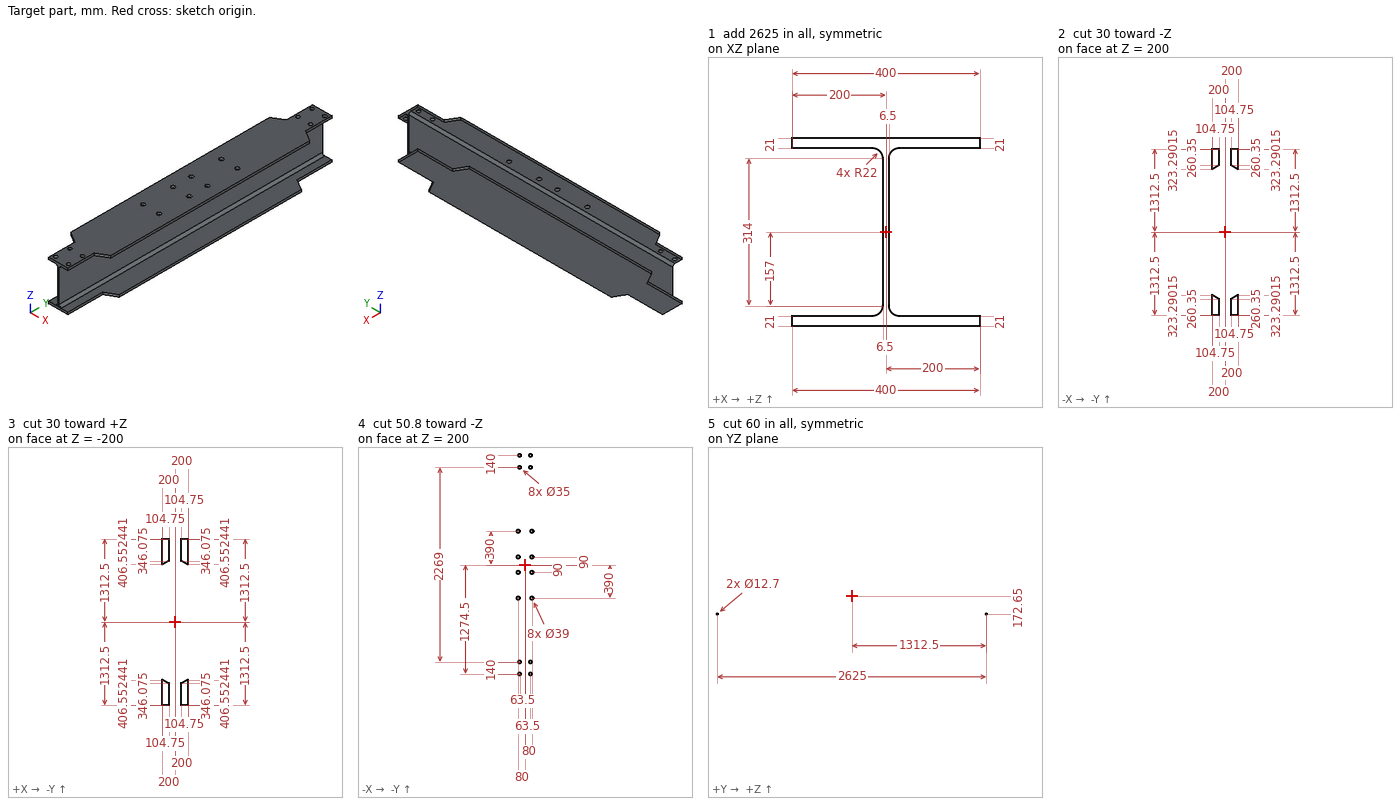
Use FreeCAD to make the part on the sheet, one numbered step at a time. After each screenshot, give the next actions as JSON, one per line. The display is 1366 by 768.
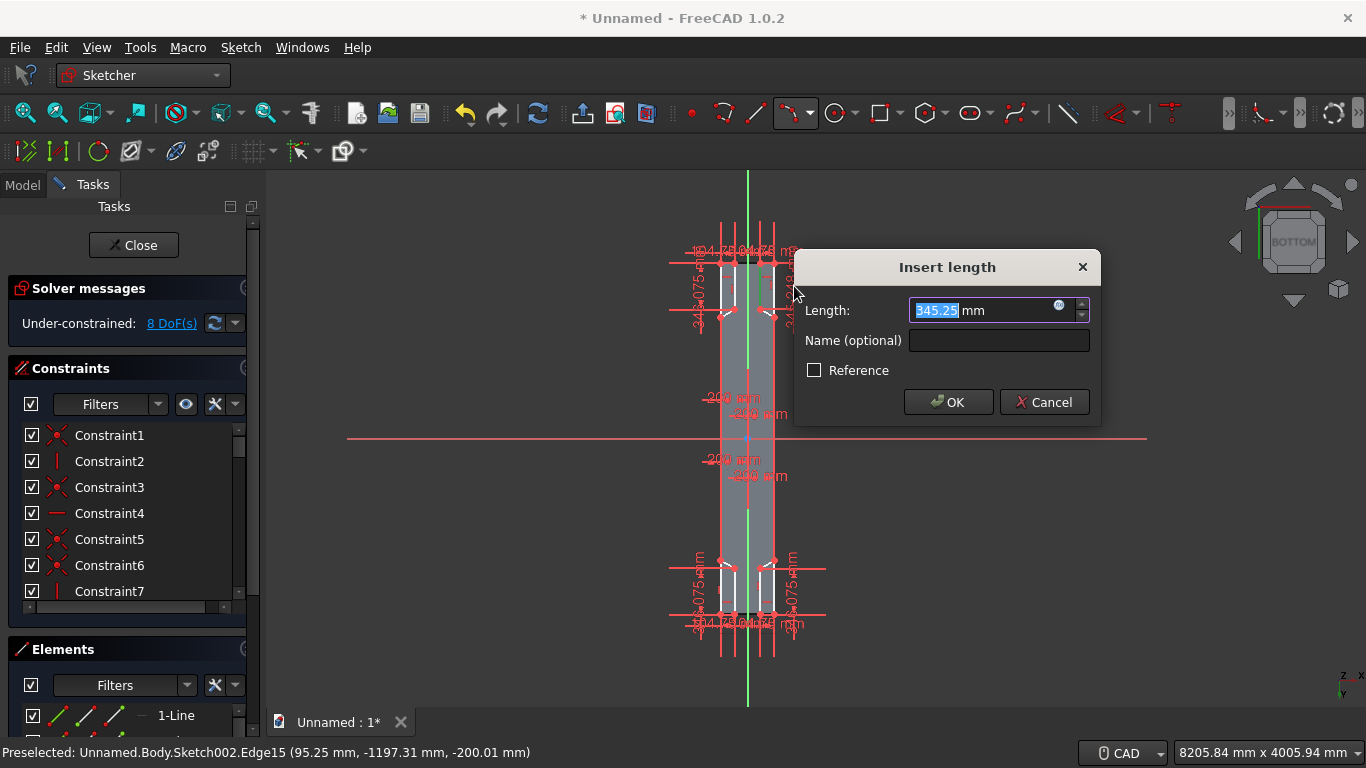
{"action": "type", "text": "346.075"}
{"action": "key", "text": "Return"}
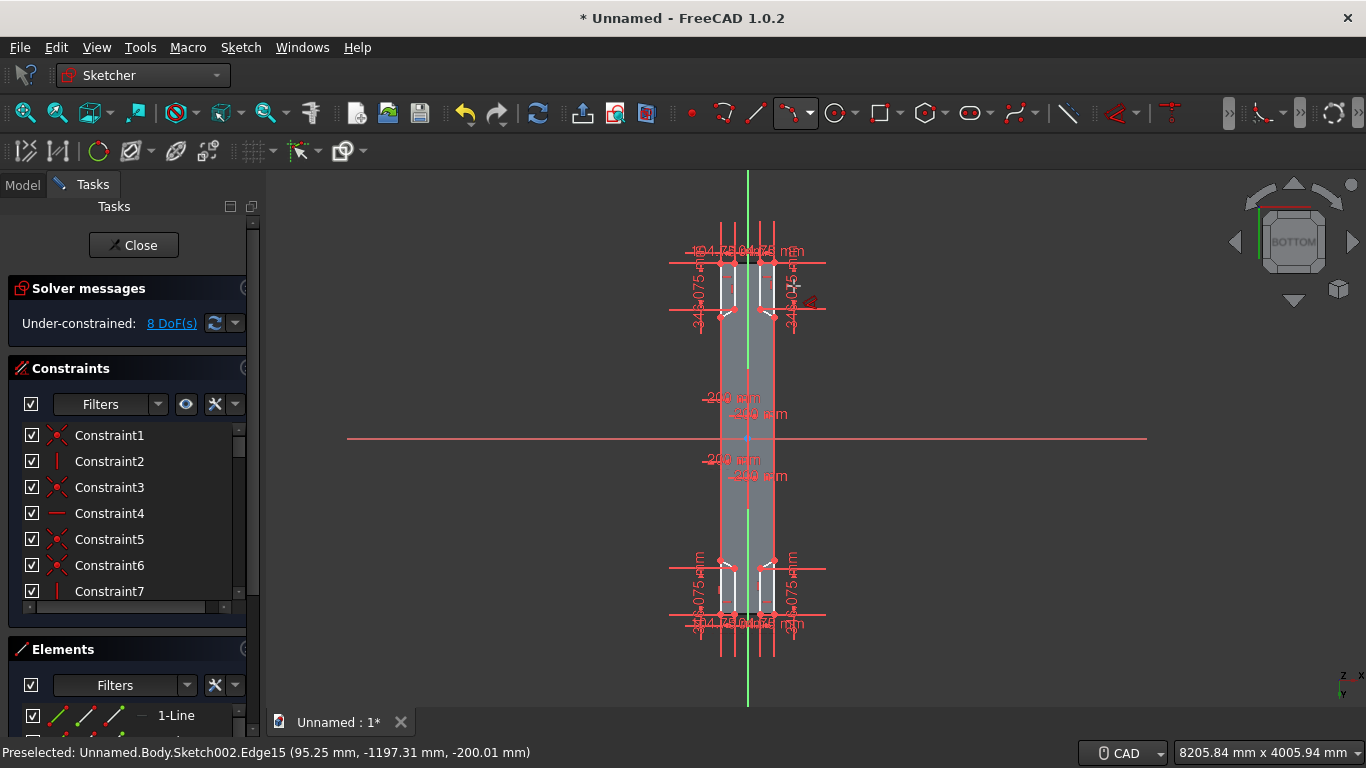
{"action": "left_click", "coordinate": [760, 615]}
{"action": "left_click", "coordinate": [794, 527]}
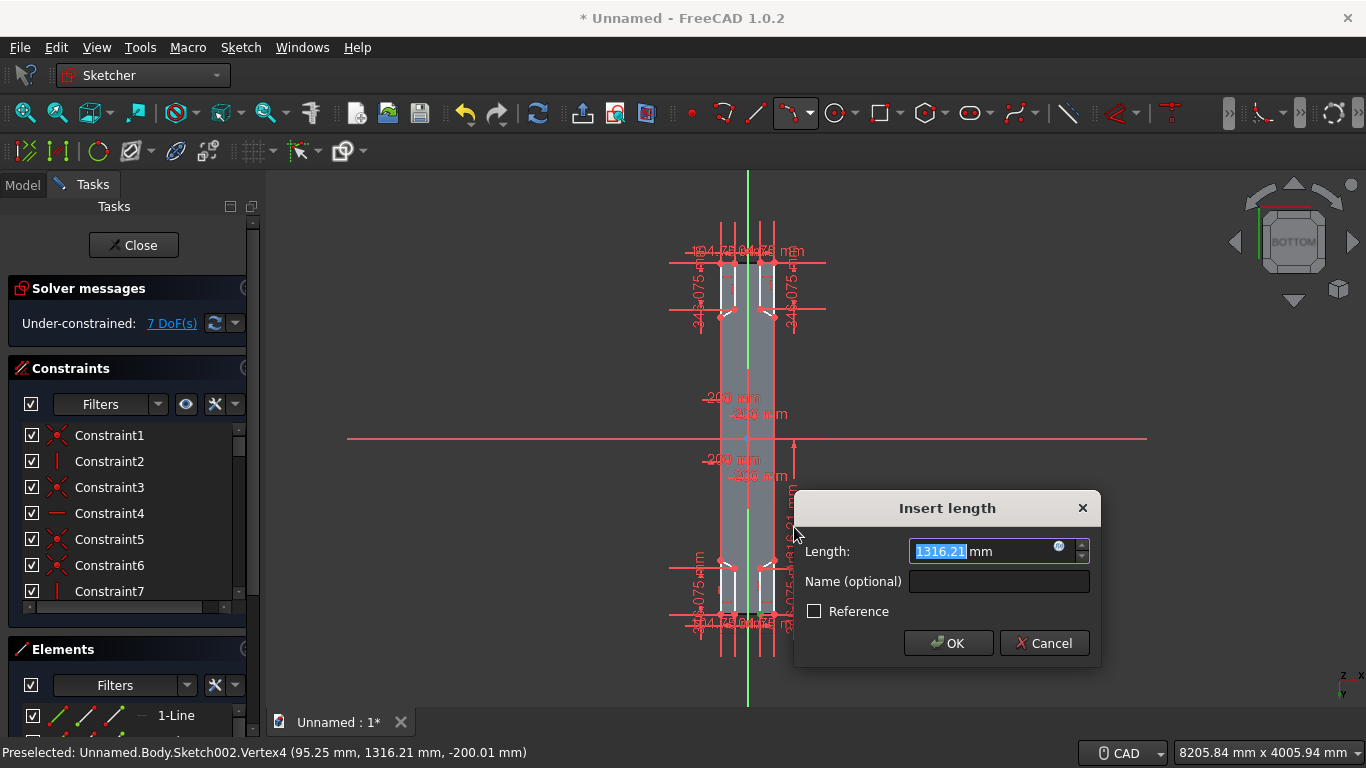
{"action": "type", "text": "1312.5"}
{"action": "key", "text": "Return"}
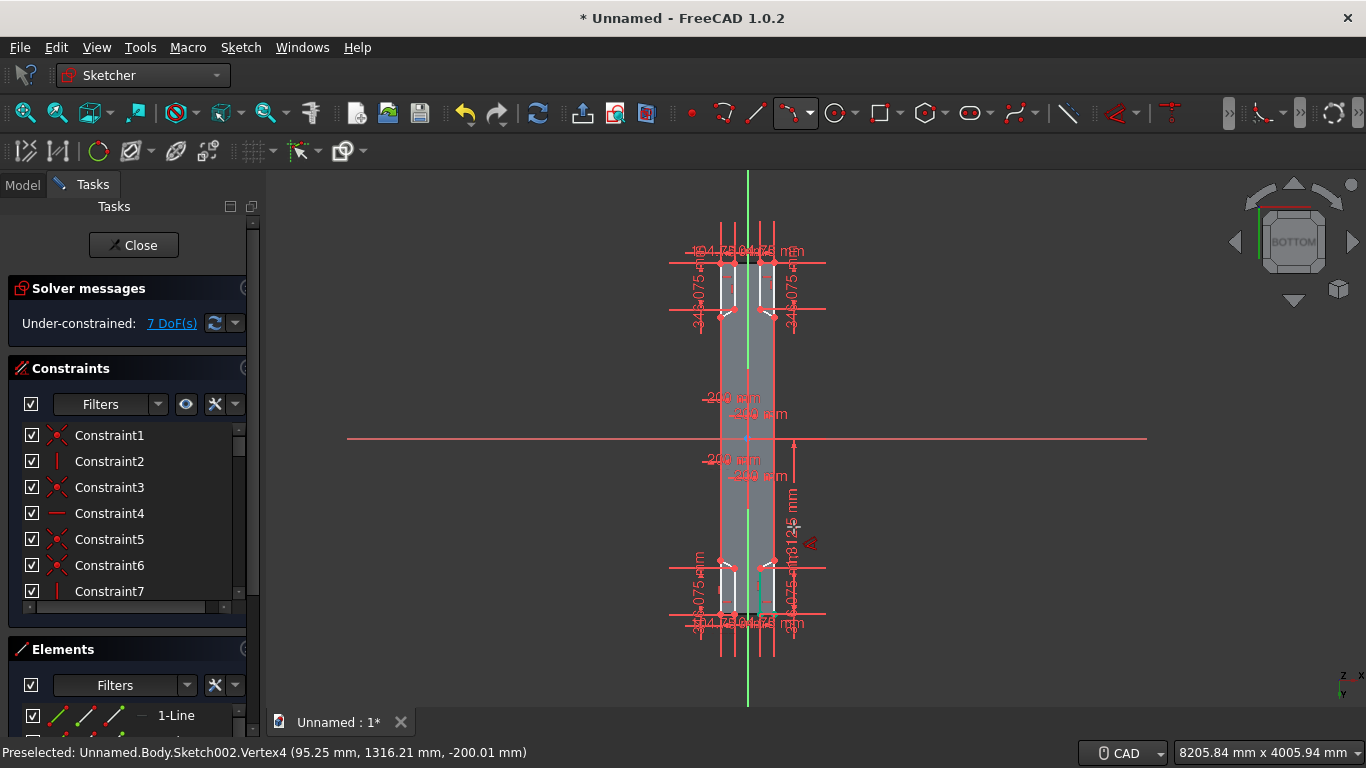
{"action": "left_click", "coordinate": [721, 615]}
{"action": "left_click", "coordinate": [687, 527]}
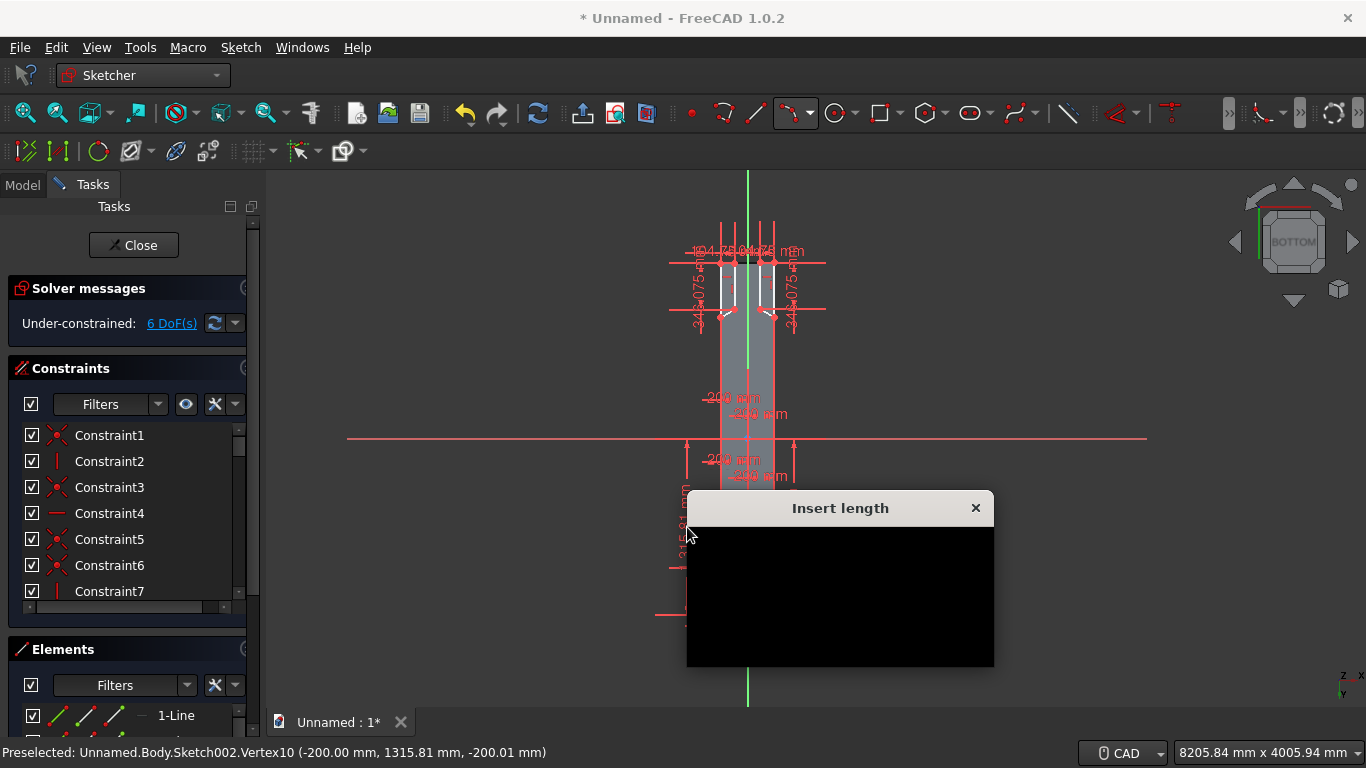
{"action": "type", "text": "1312.5"}
{"action": "key", "text": "Return"}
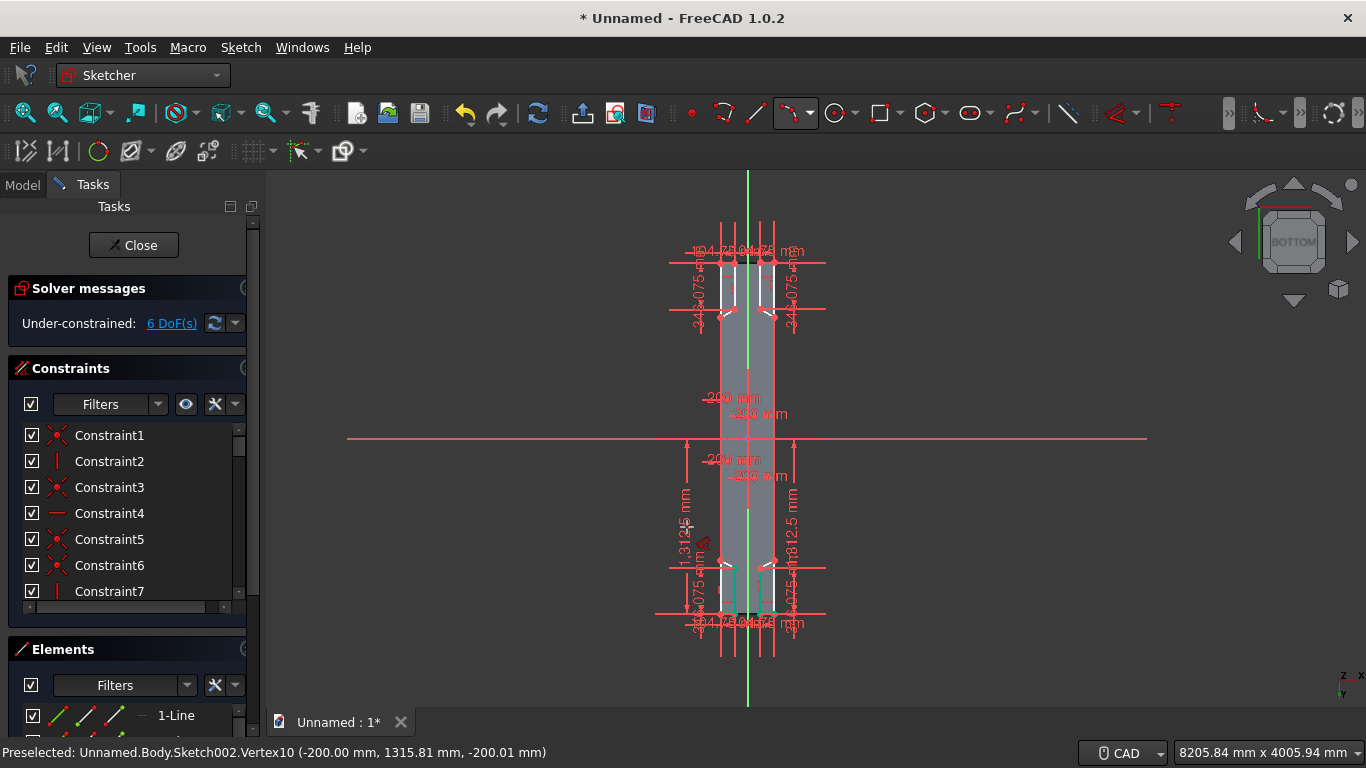
{"action": "left_click", "coordinate": [735, 263]}
{"action": "left_click", "coordinate": [701, 351]}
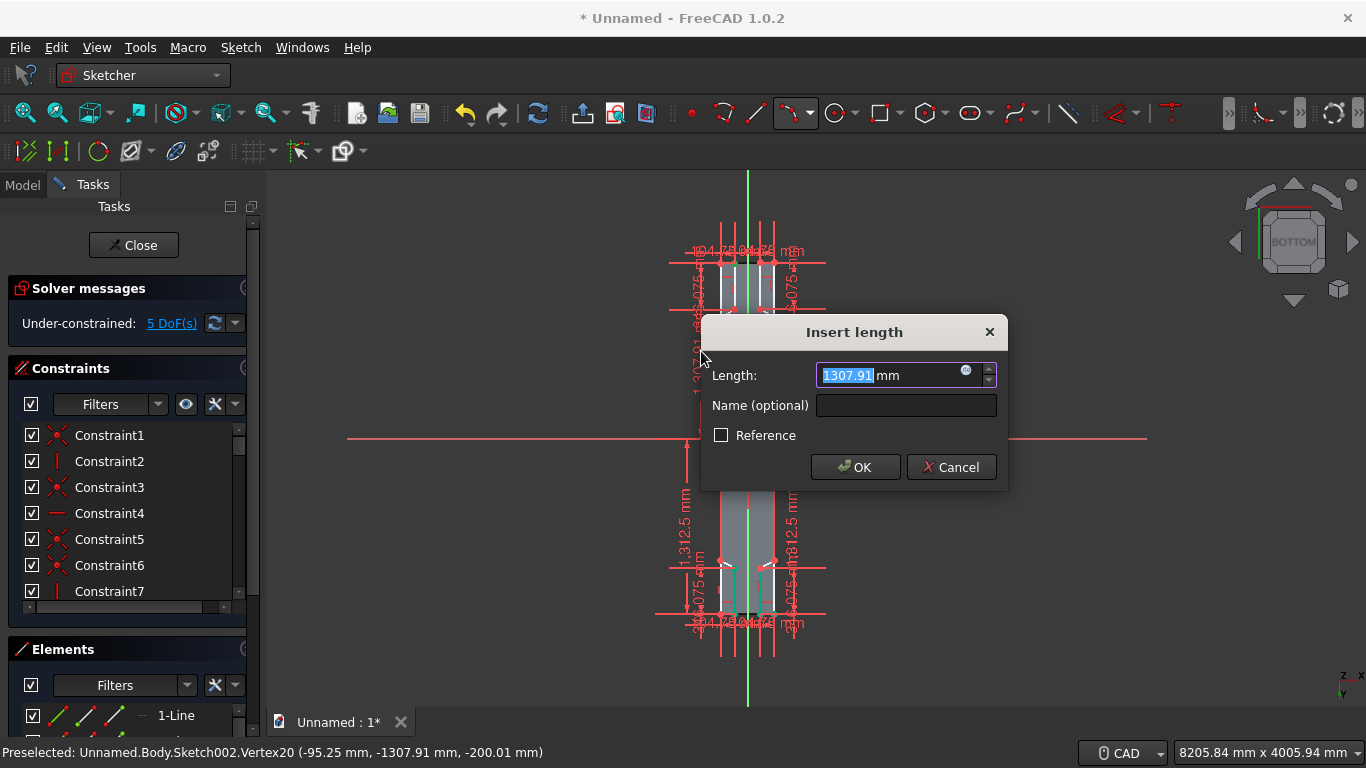
{"action": "type", "text": "1312.5"}
{"action": "key", "text": "Return"}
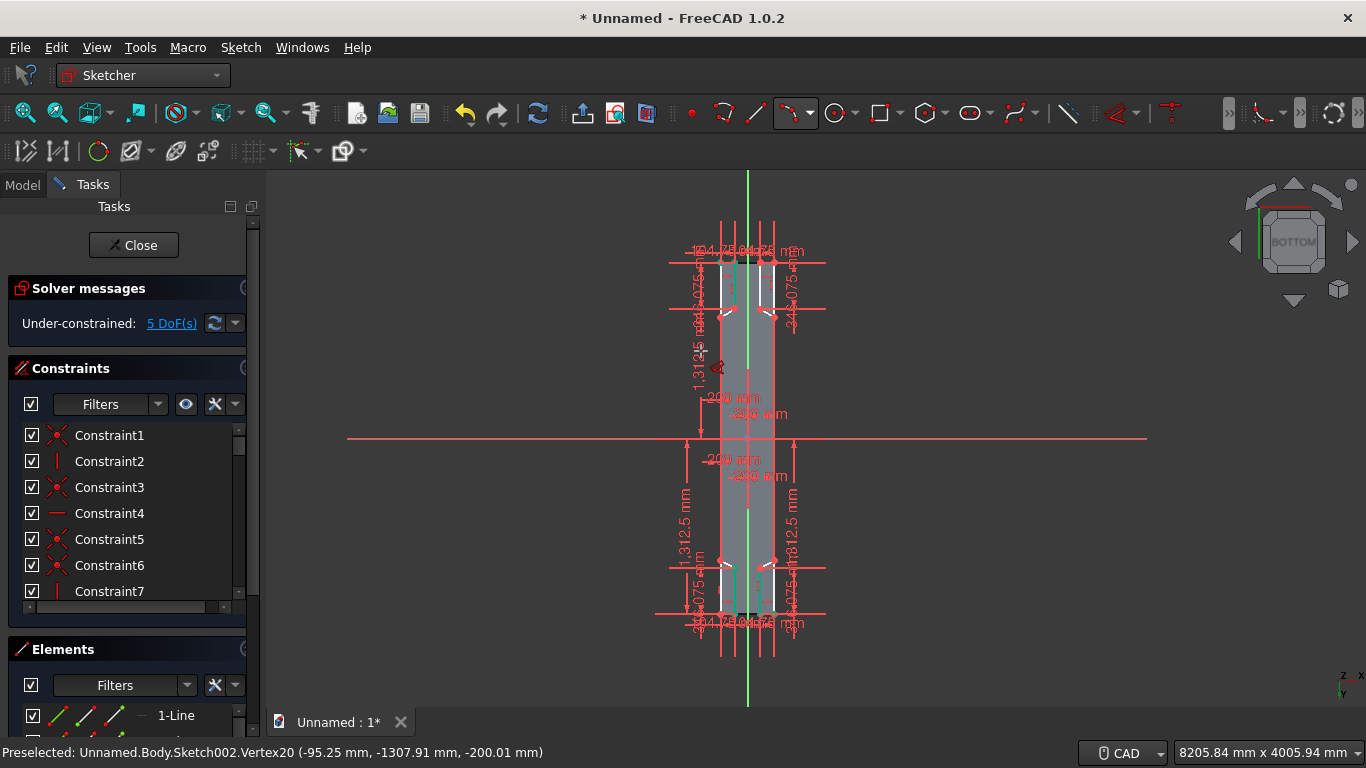
{"action": "left_click", "coordinate": [774, 263]}
{"action": "left_click", "coordinate": [808, 351]}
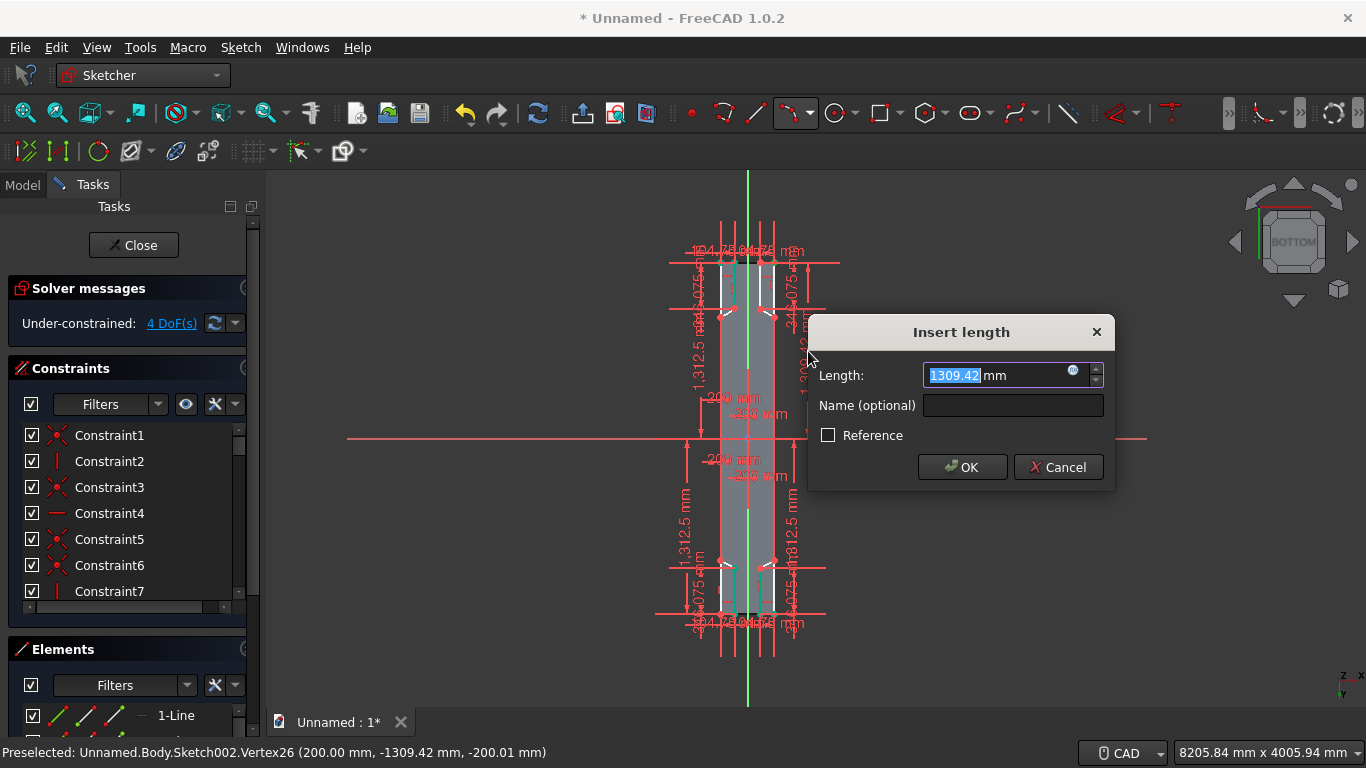
{"action": "type", "text": "1312.5"}
{"action": "key", "text": "Return"}